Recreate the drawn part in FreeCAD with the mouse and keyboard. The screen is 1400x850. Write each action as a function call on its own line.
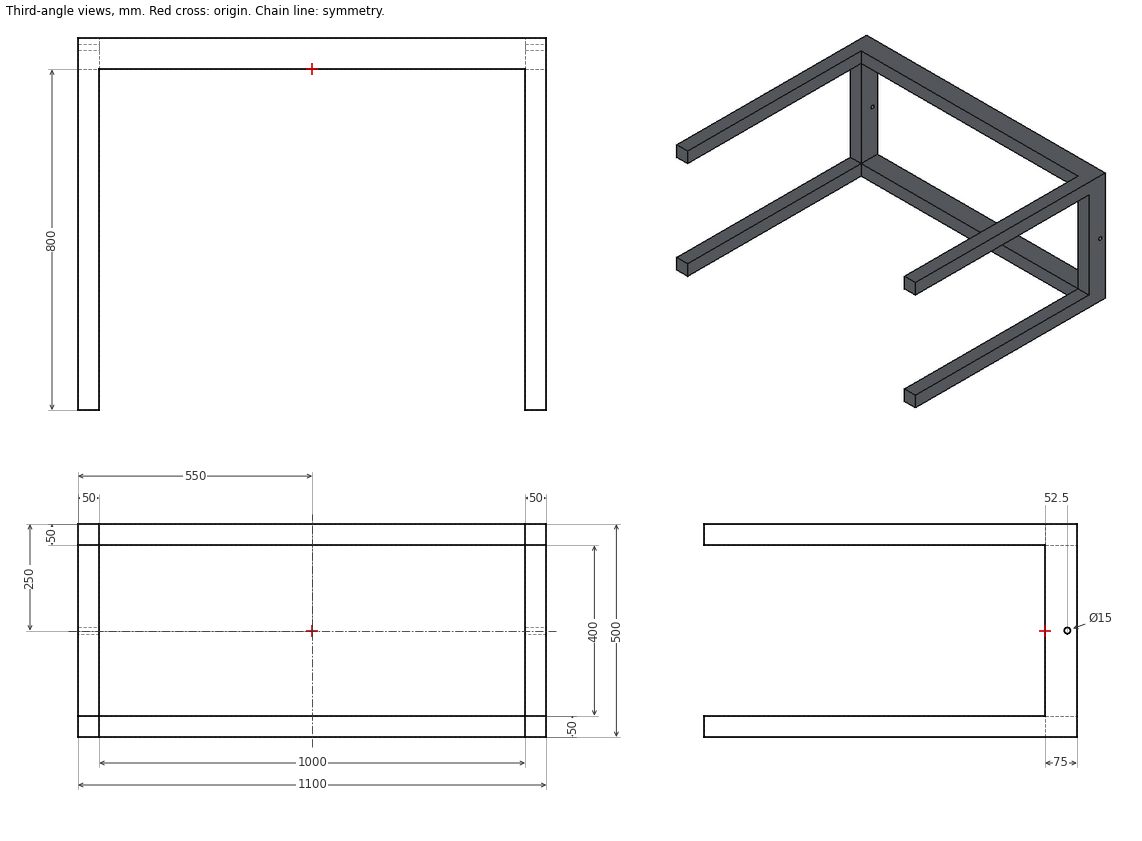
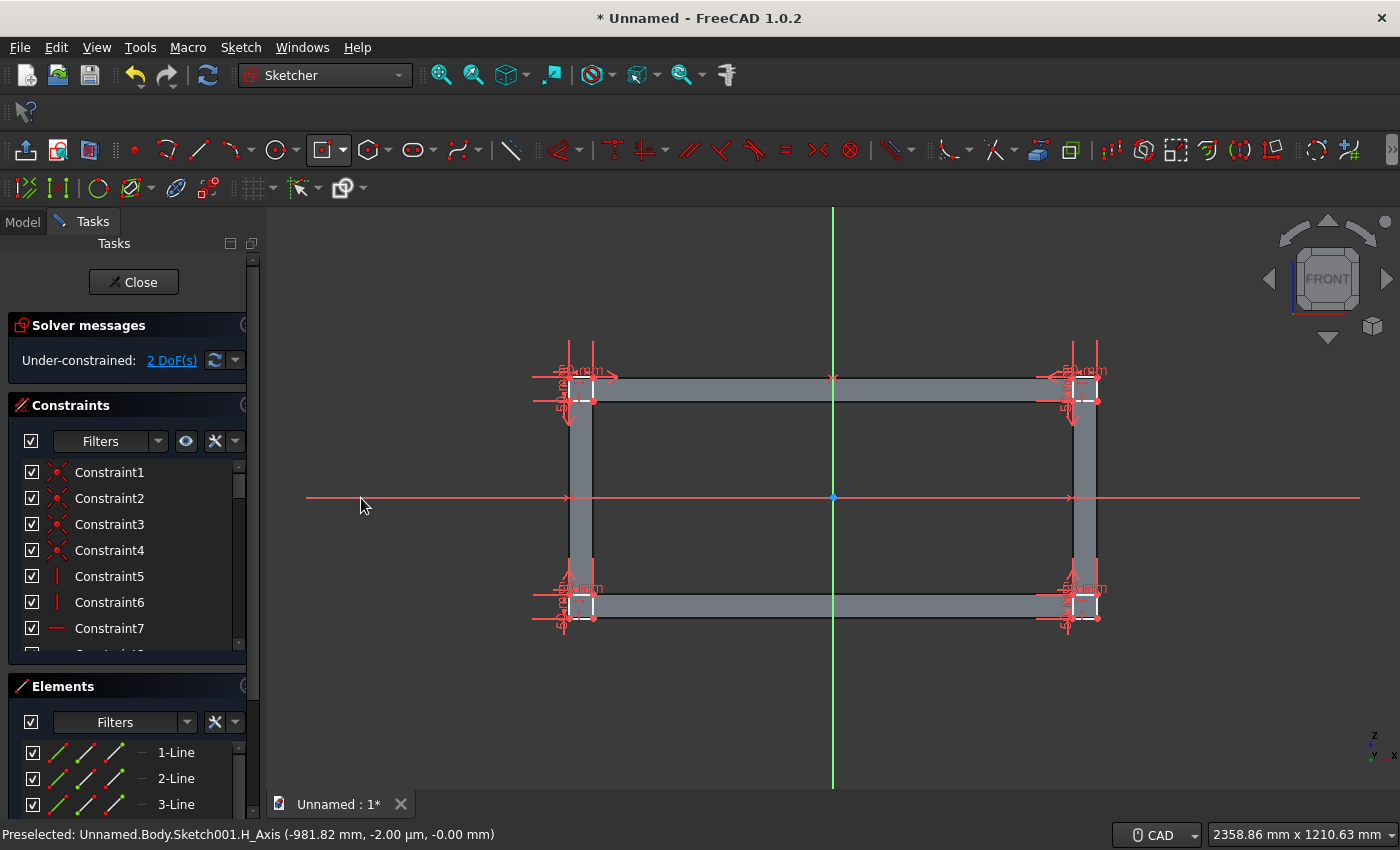
click(558, 150)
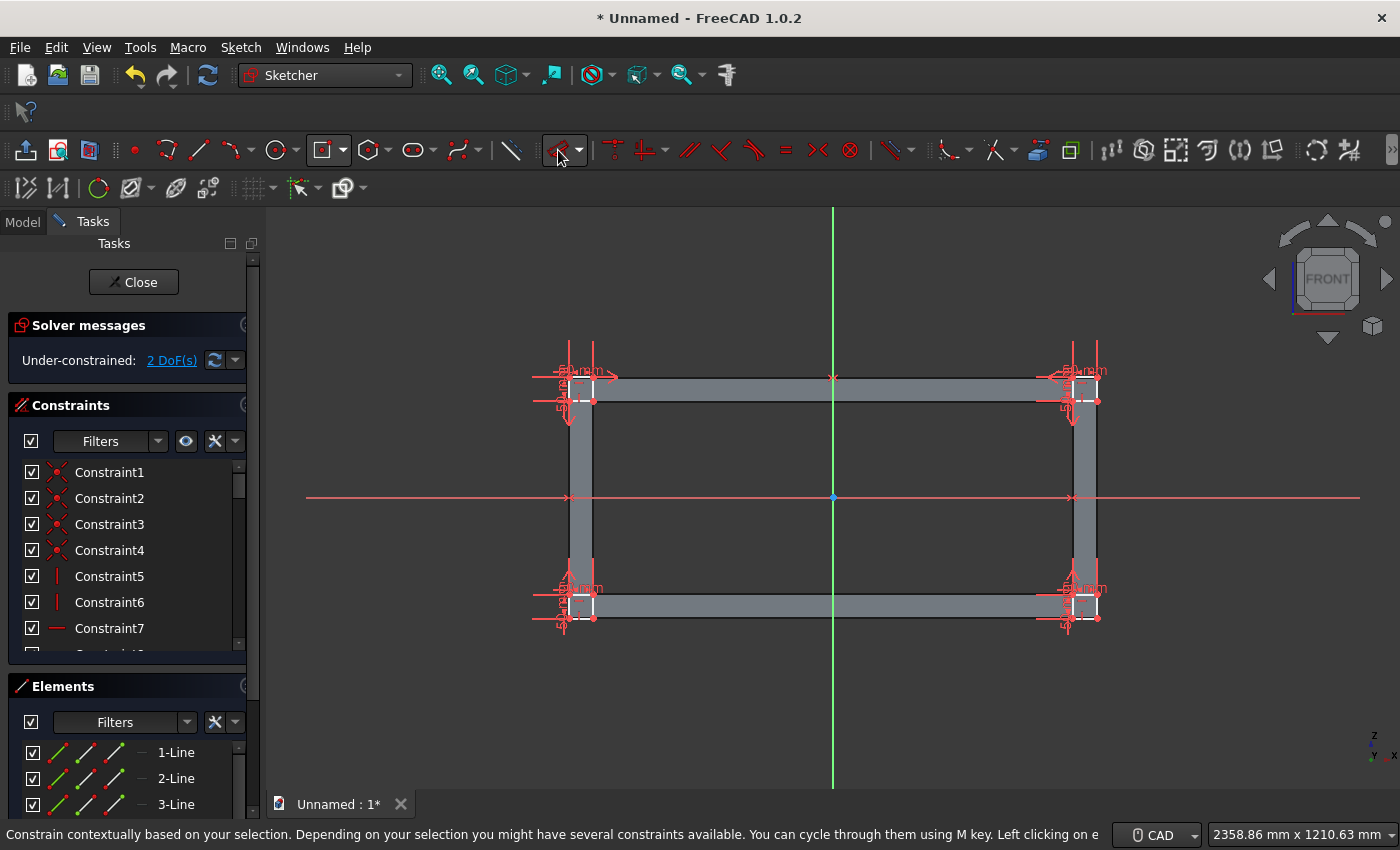
click(569, 377)
click(701, 343)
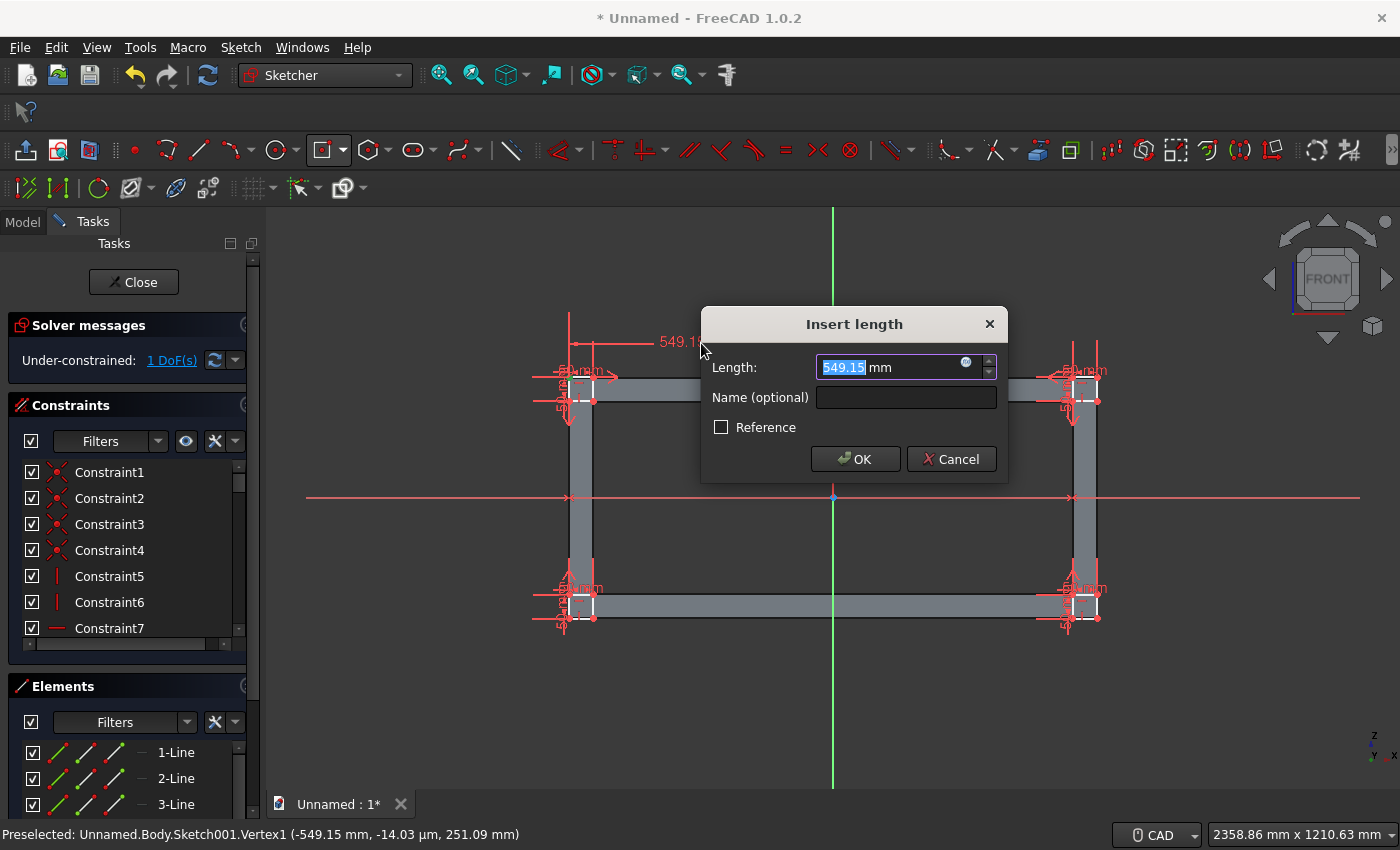
text(550)
key(Return)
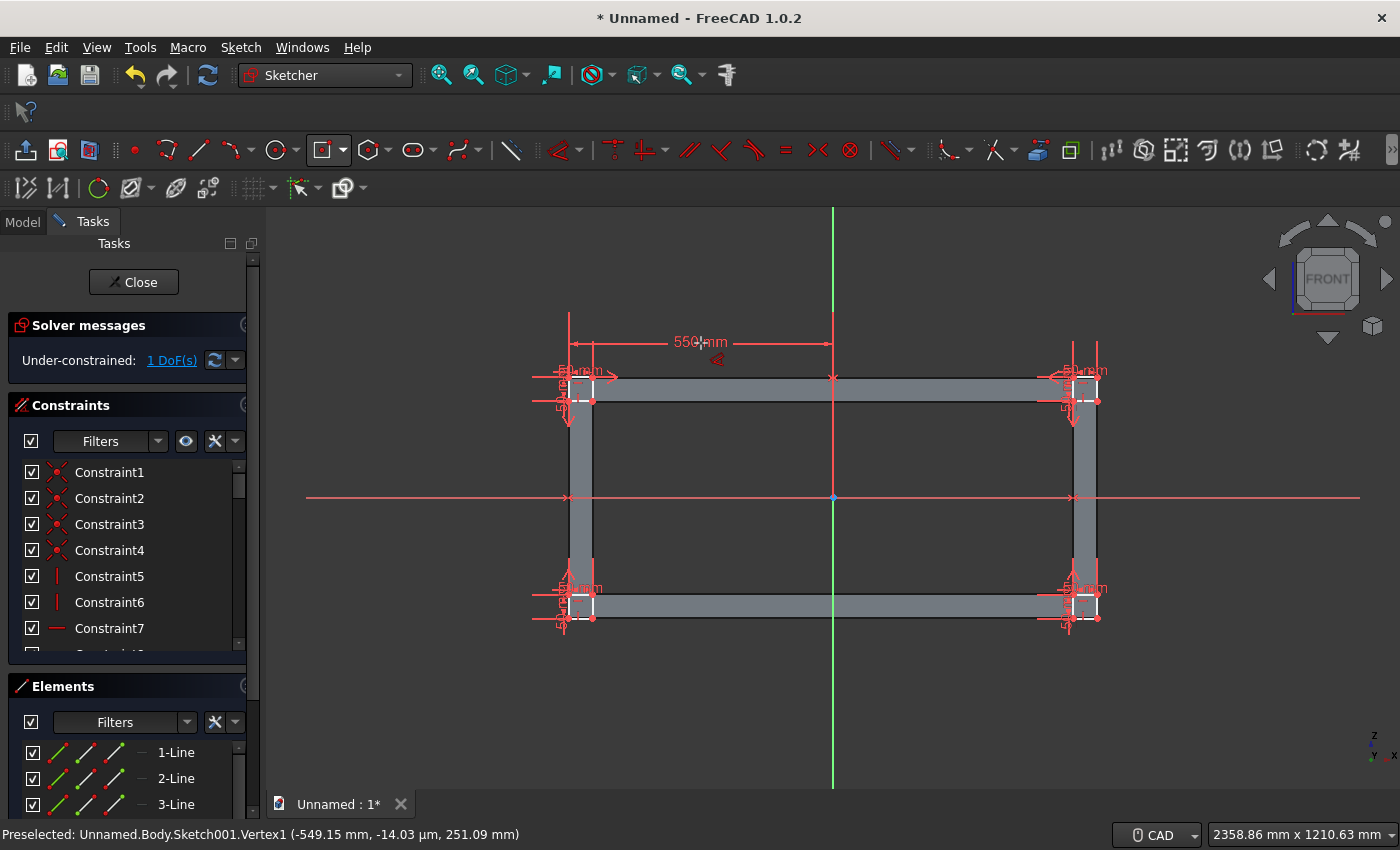
click(569, 377)
click(535, 438)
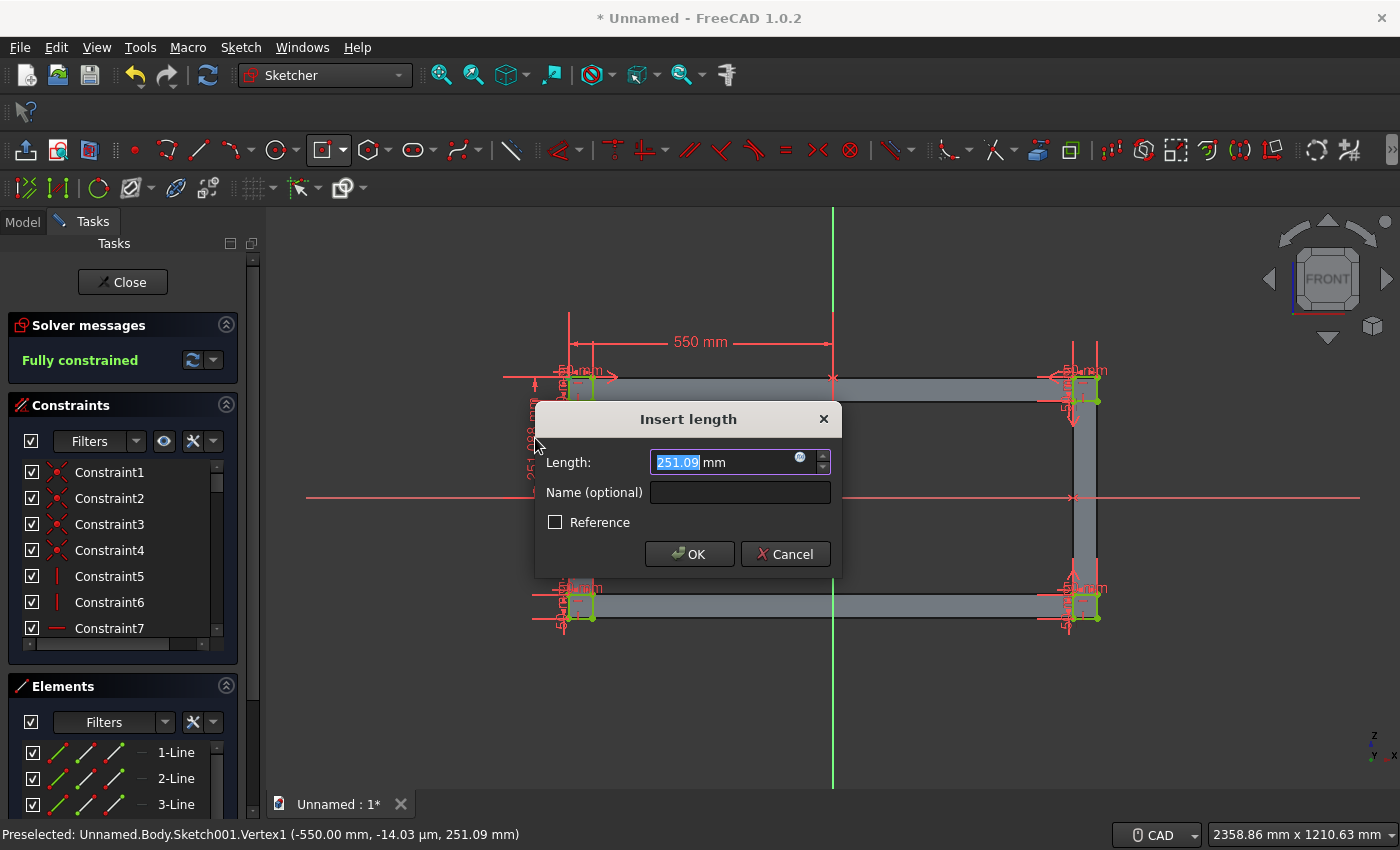
text(250)
key(Return)
key(Escape)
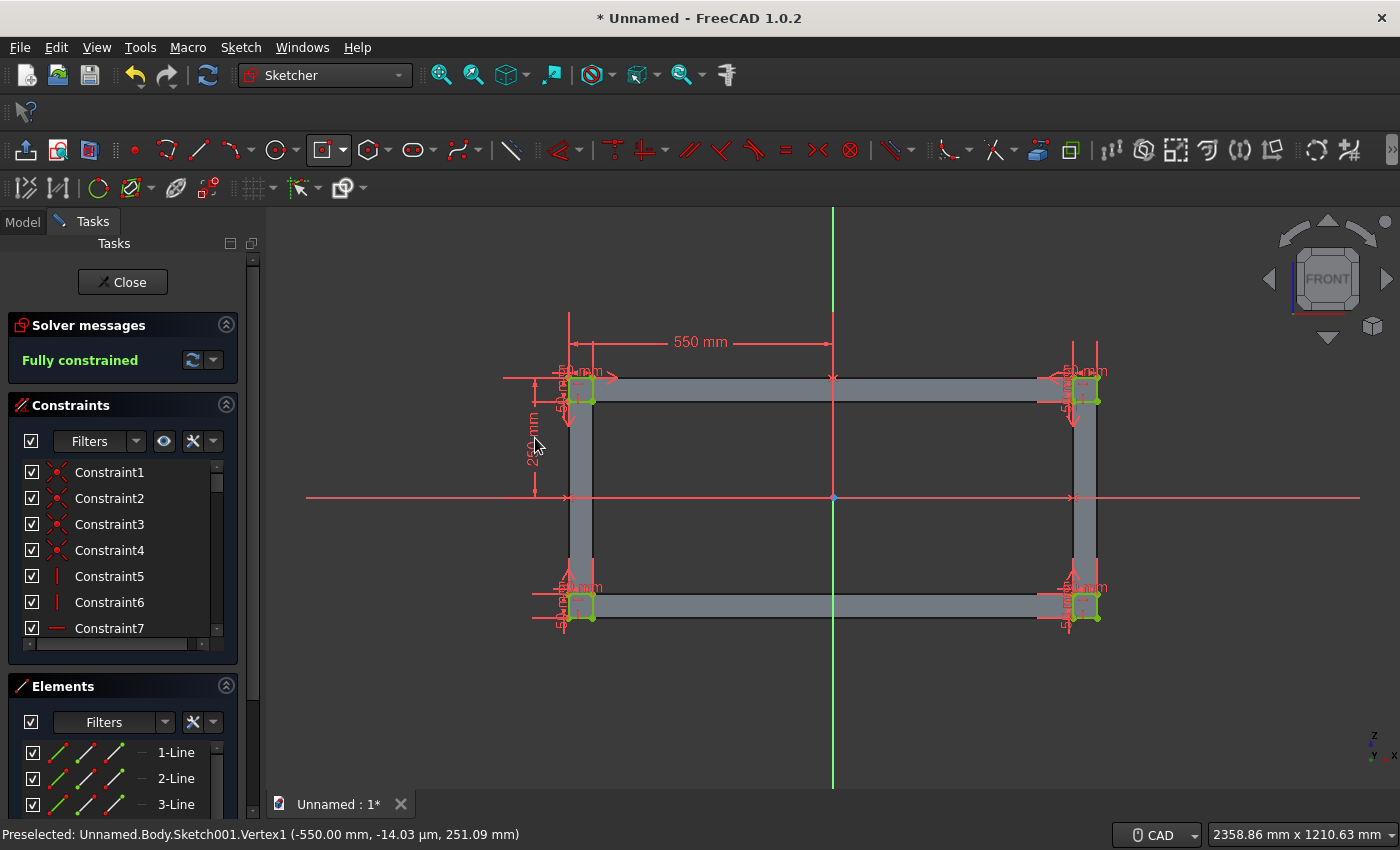
click(123, 282)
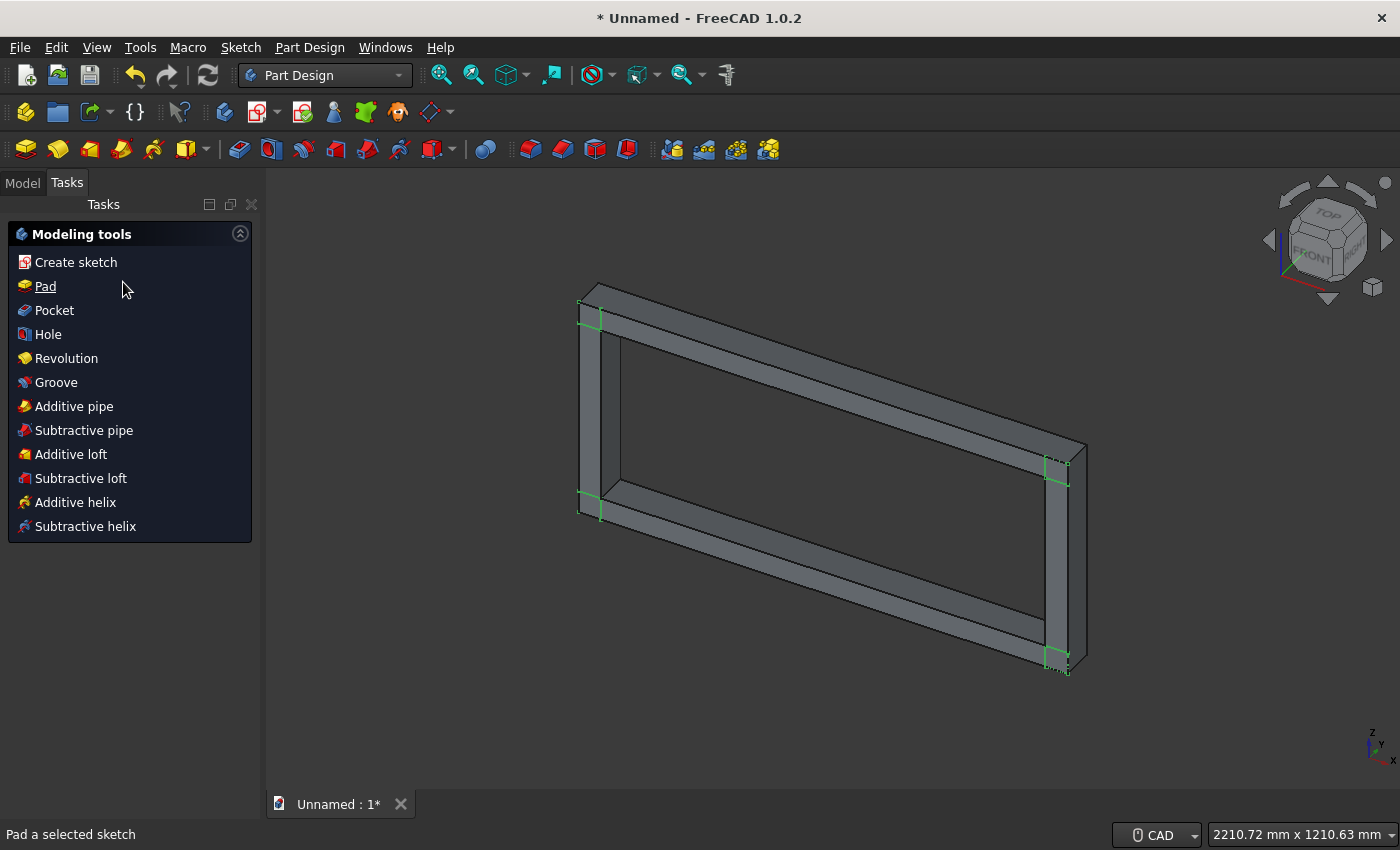
click(26, 150)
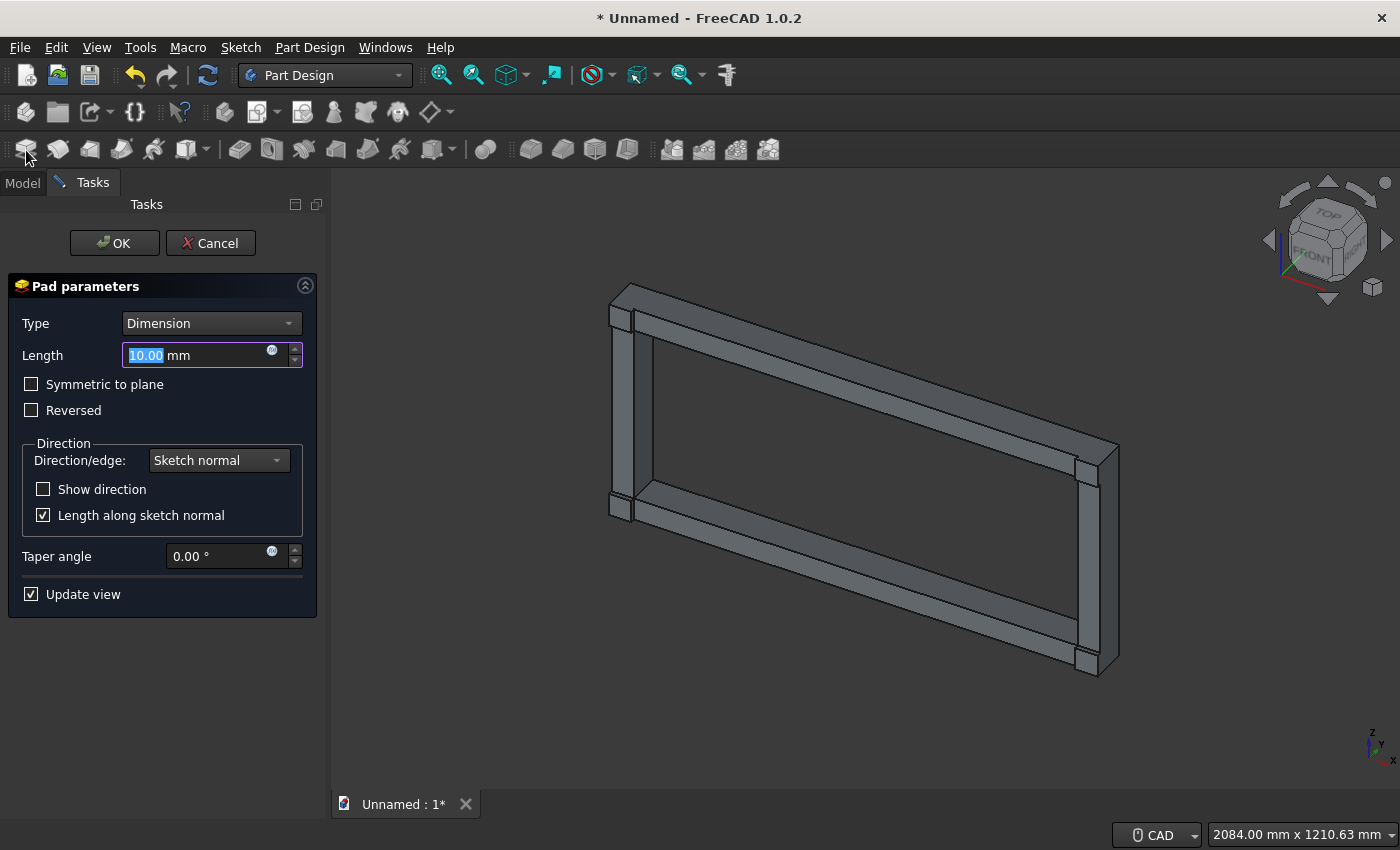
text(800)
key(Tab)